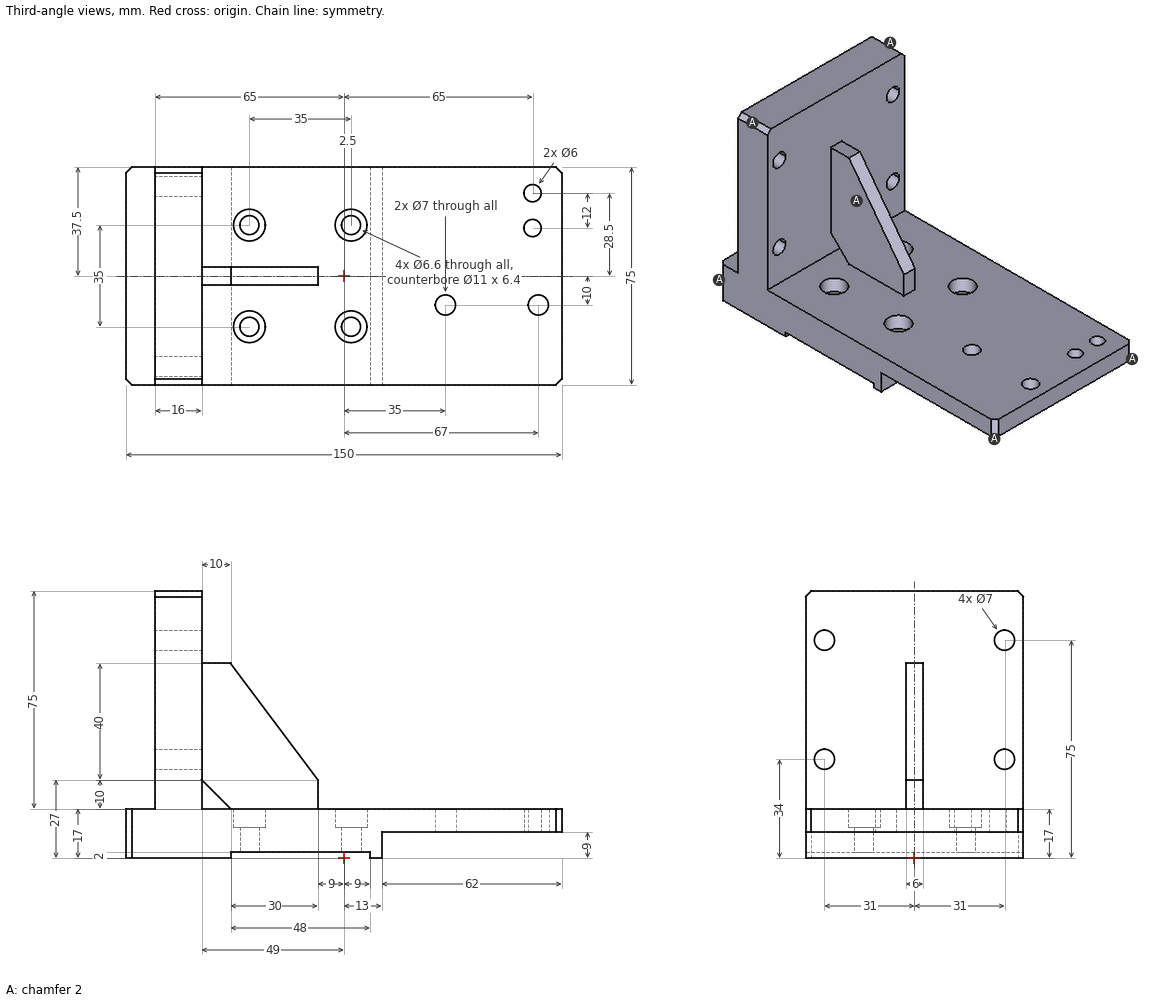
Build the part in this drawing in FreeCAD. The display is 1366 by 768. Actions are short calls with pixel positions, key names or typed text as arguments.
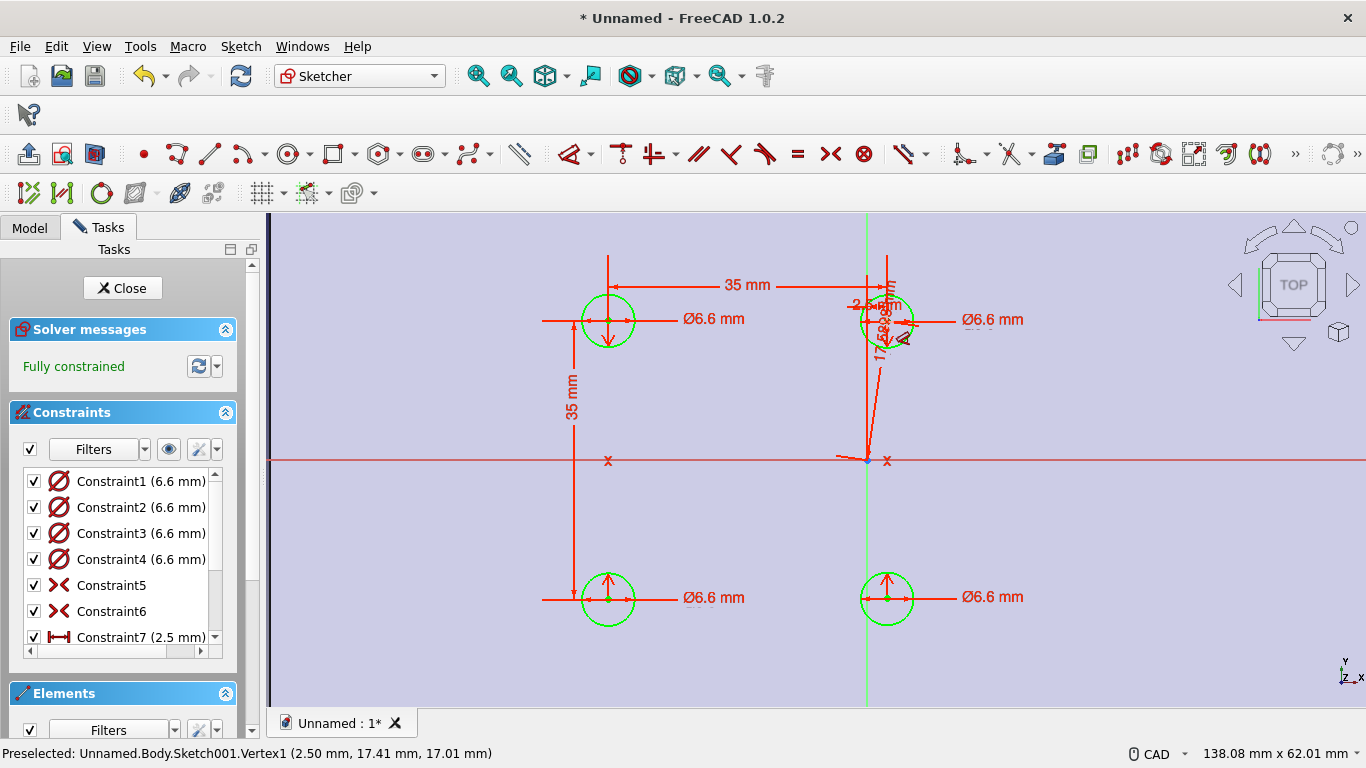
click(608, 600)
click(921, 397)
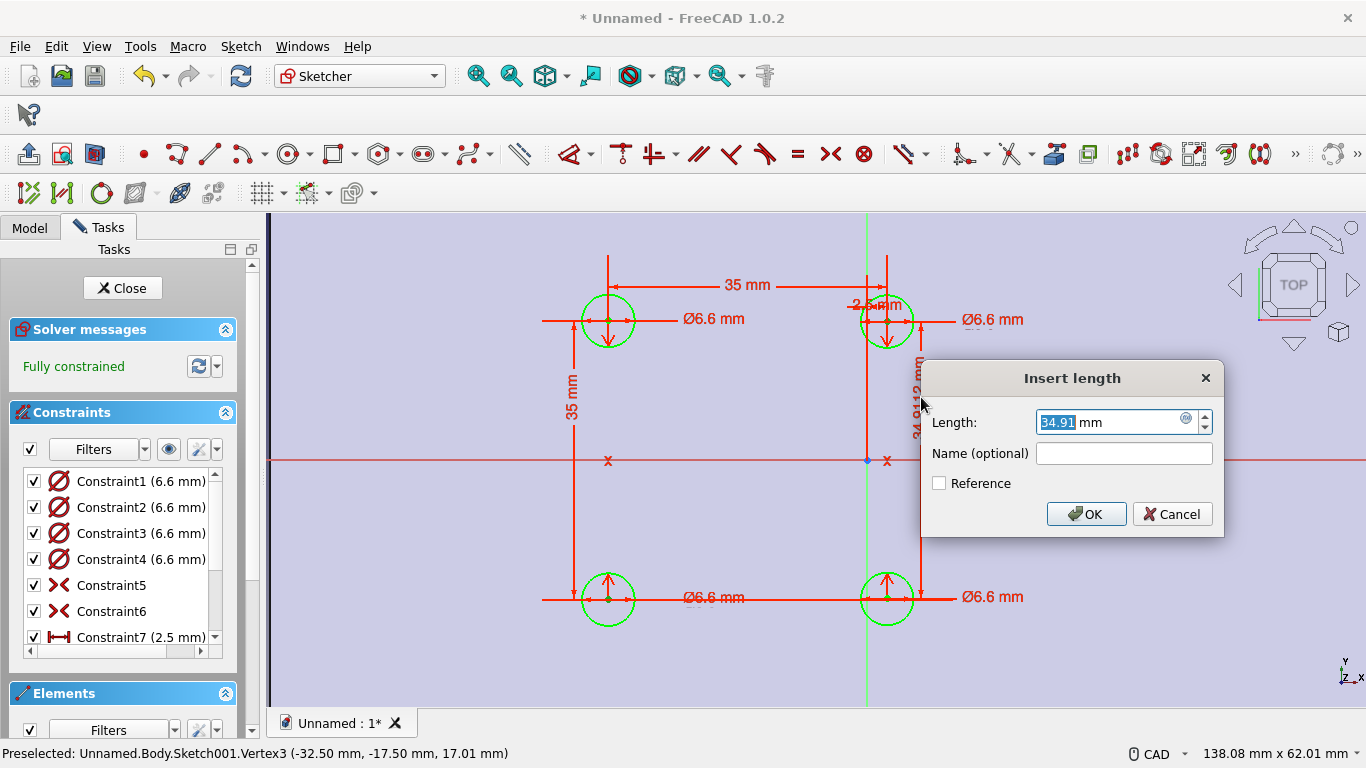
text(35)
key(Return)
key(Escape)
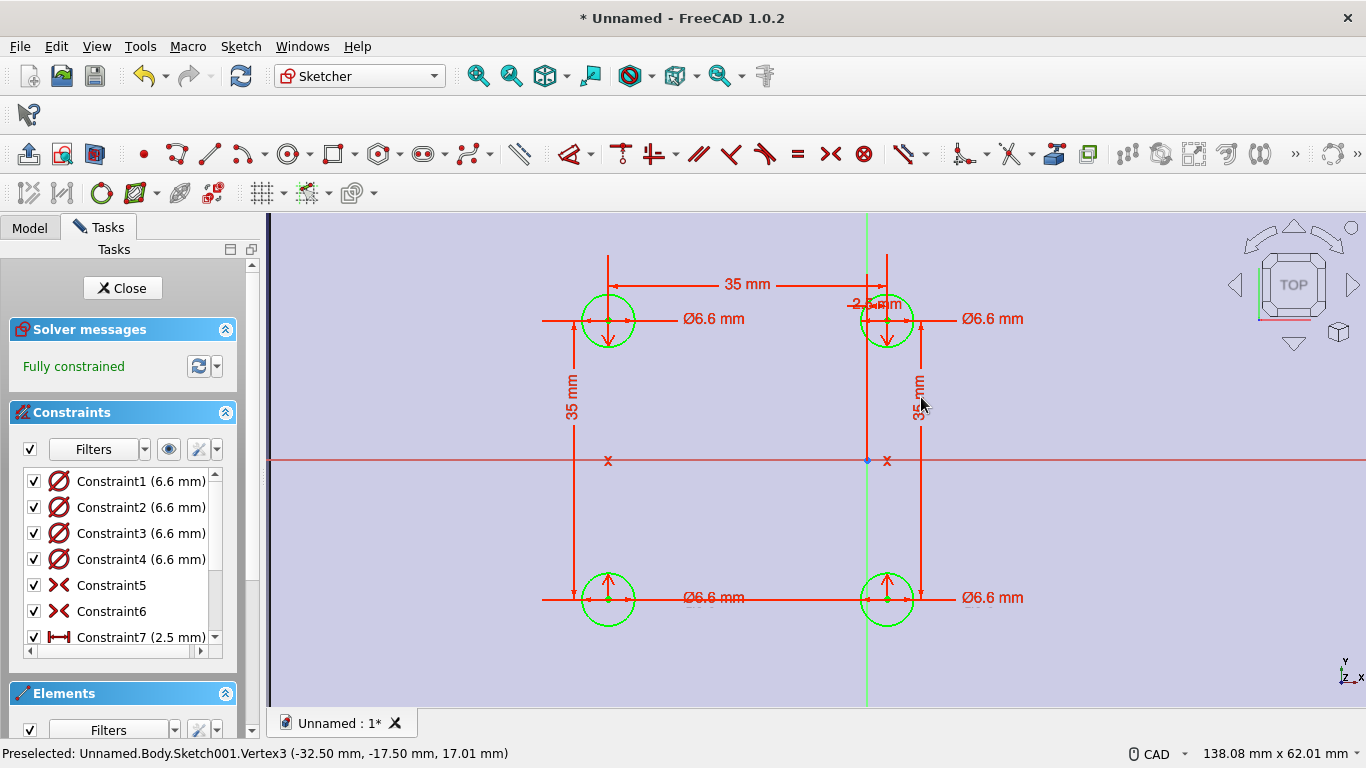
click(123, 288)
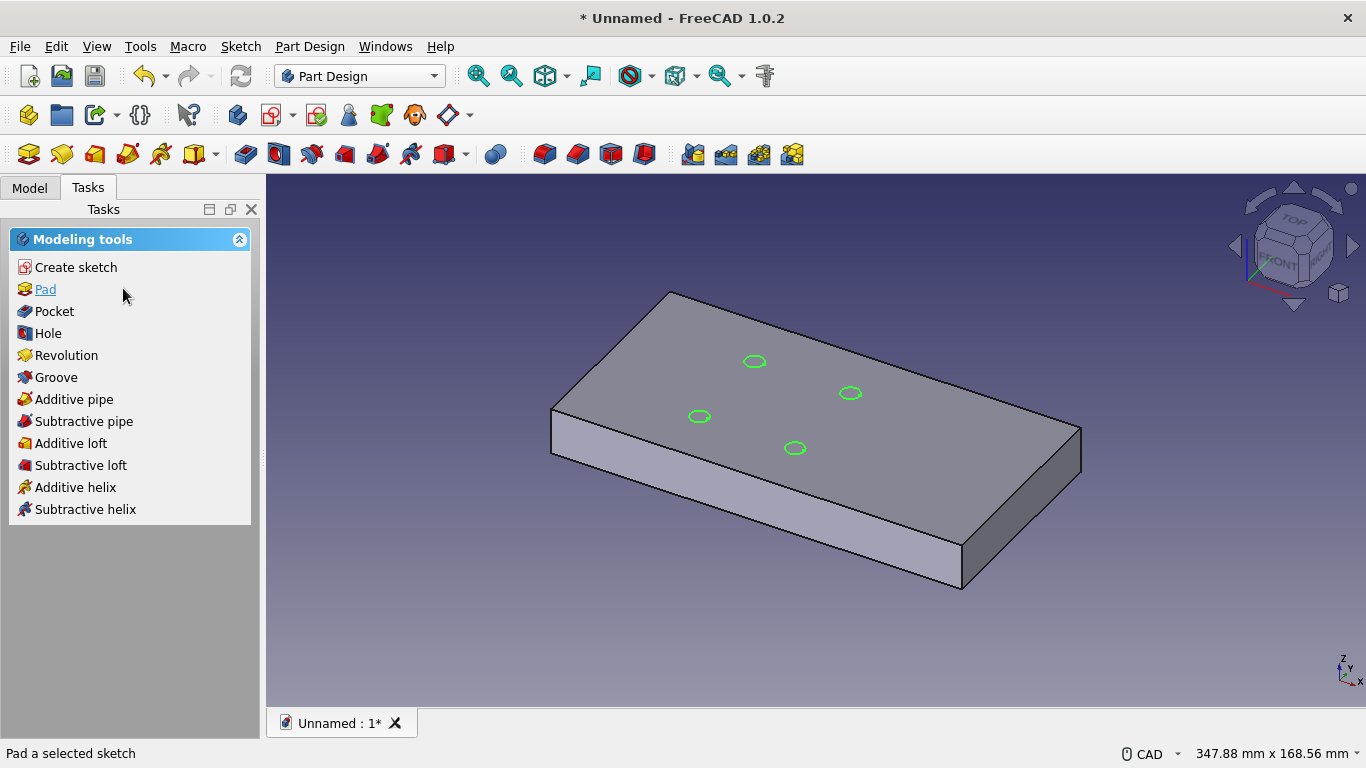
click(279, 154)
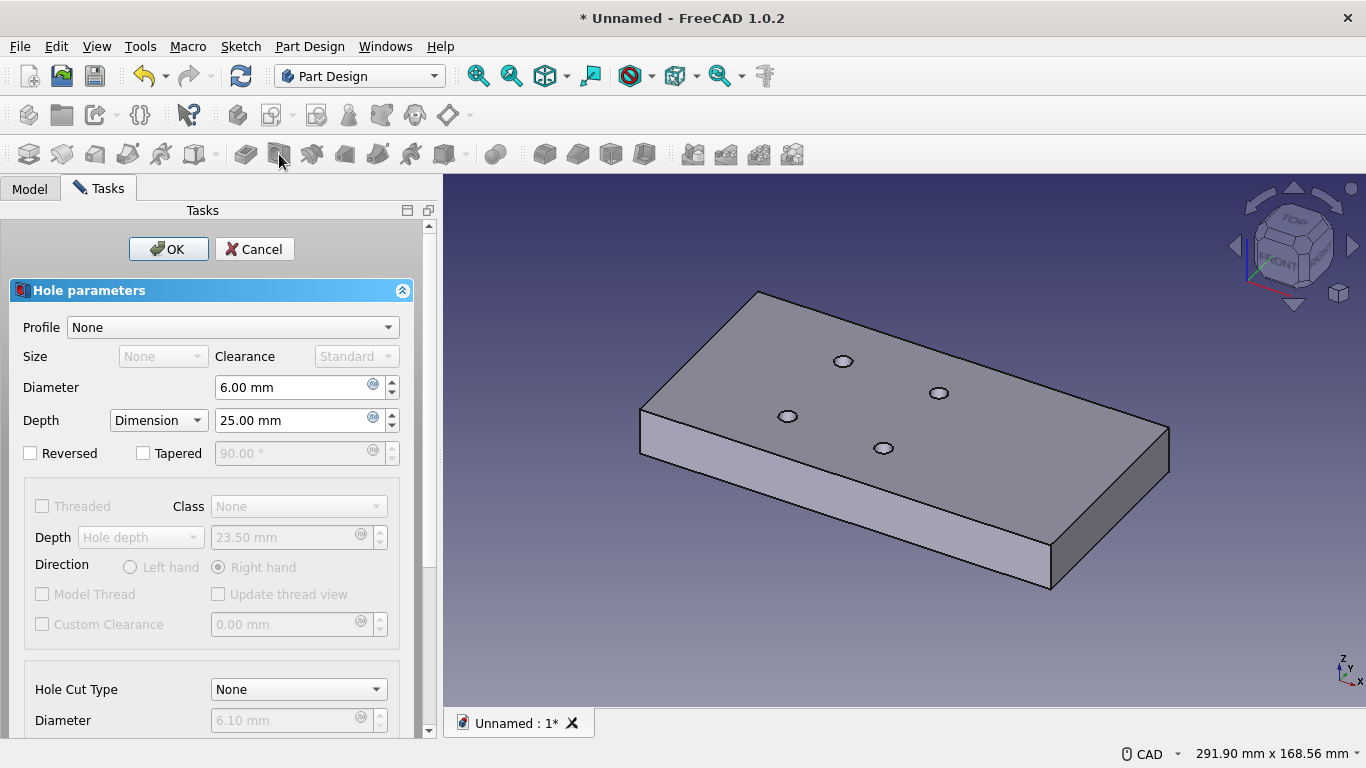
triple_click(300, 388)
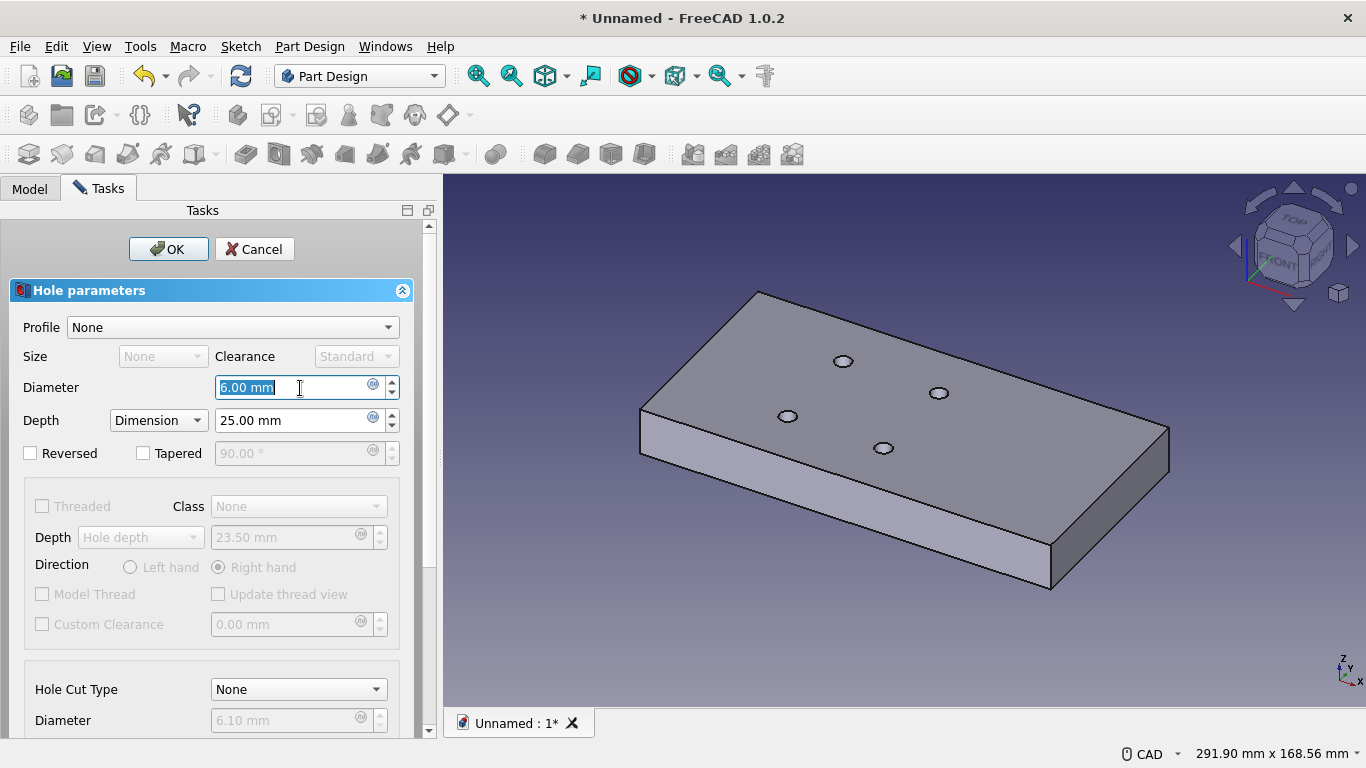
text(6.6)
key(Tab)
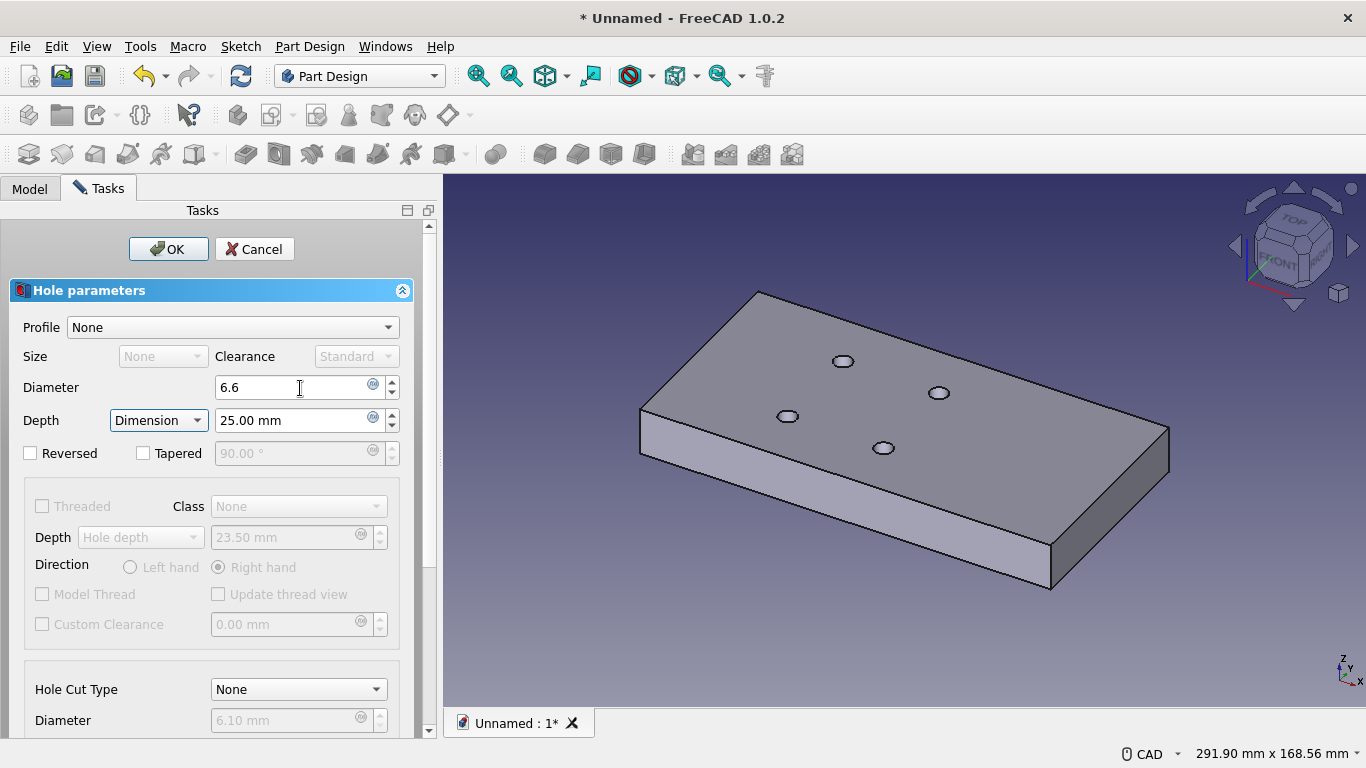
click(160, 420)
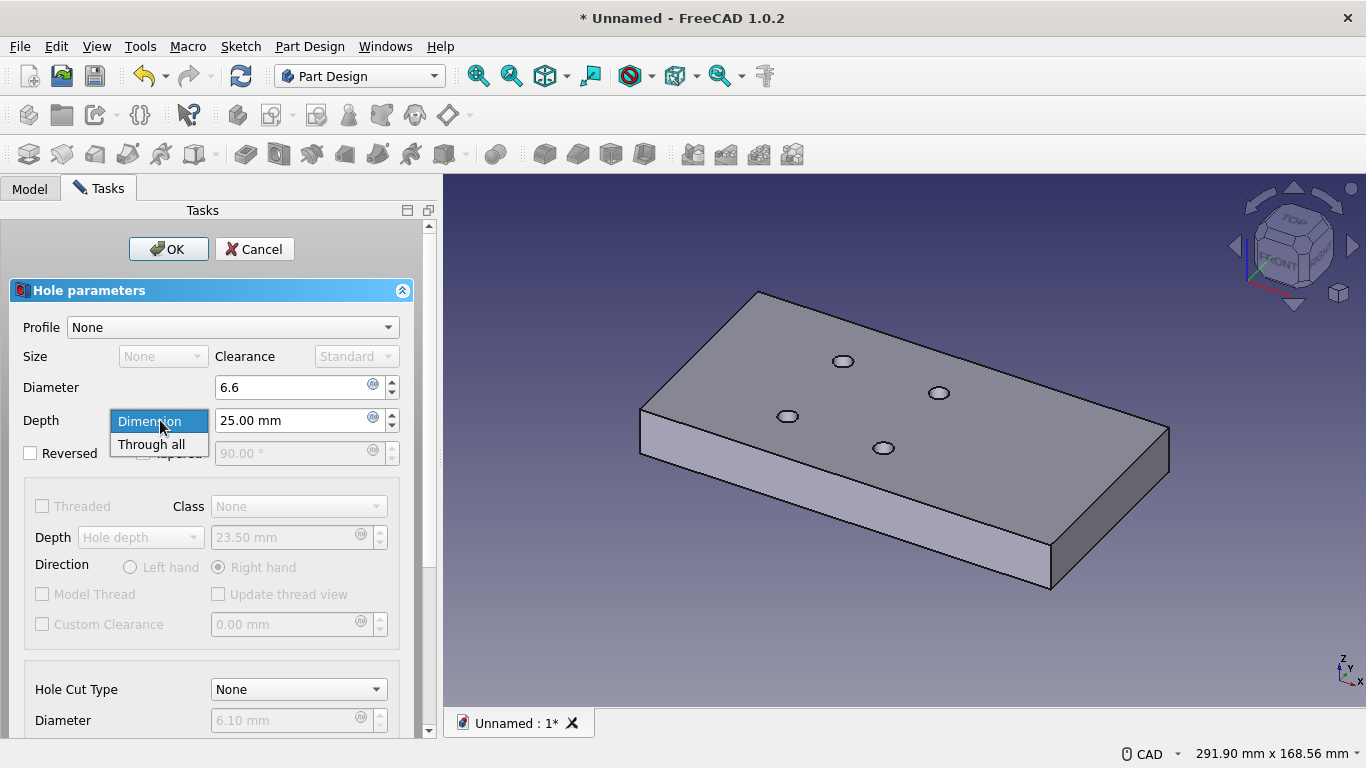
click(158, 444)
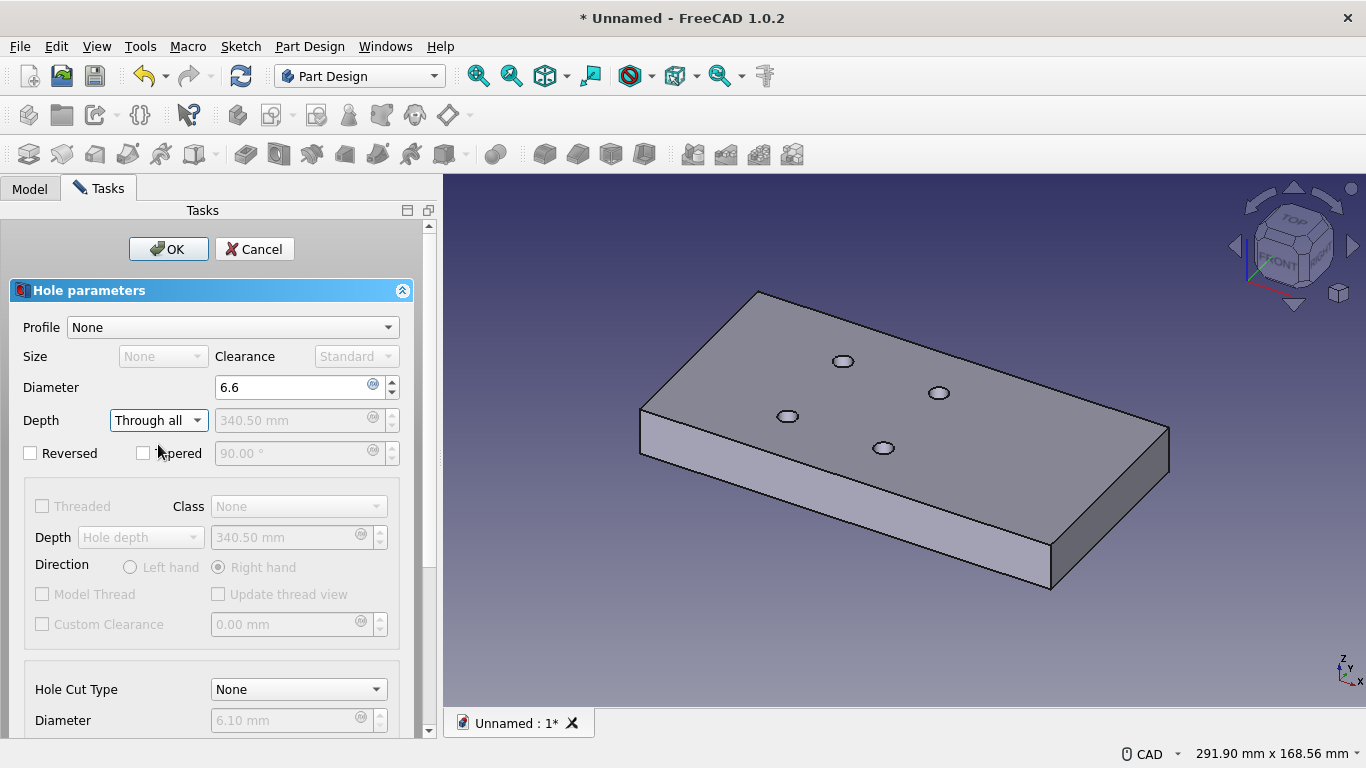
click(300, 690)